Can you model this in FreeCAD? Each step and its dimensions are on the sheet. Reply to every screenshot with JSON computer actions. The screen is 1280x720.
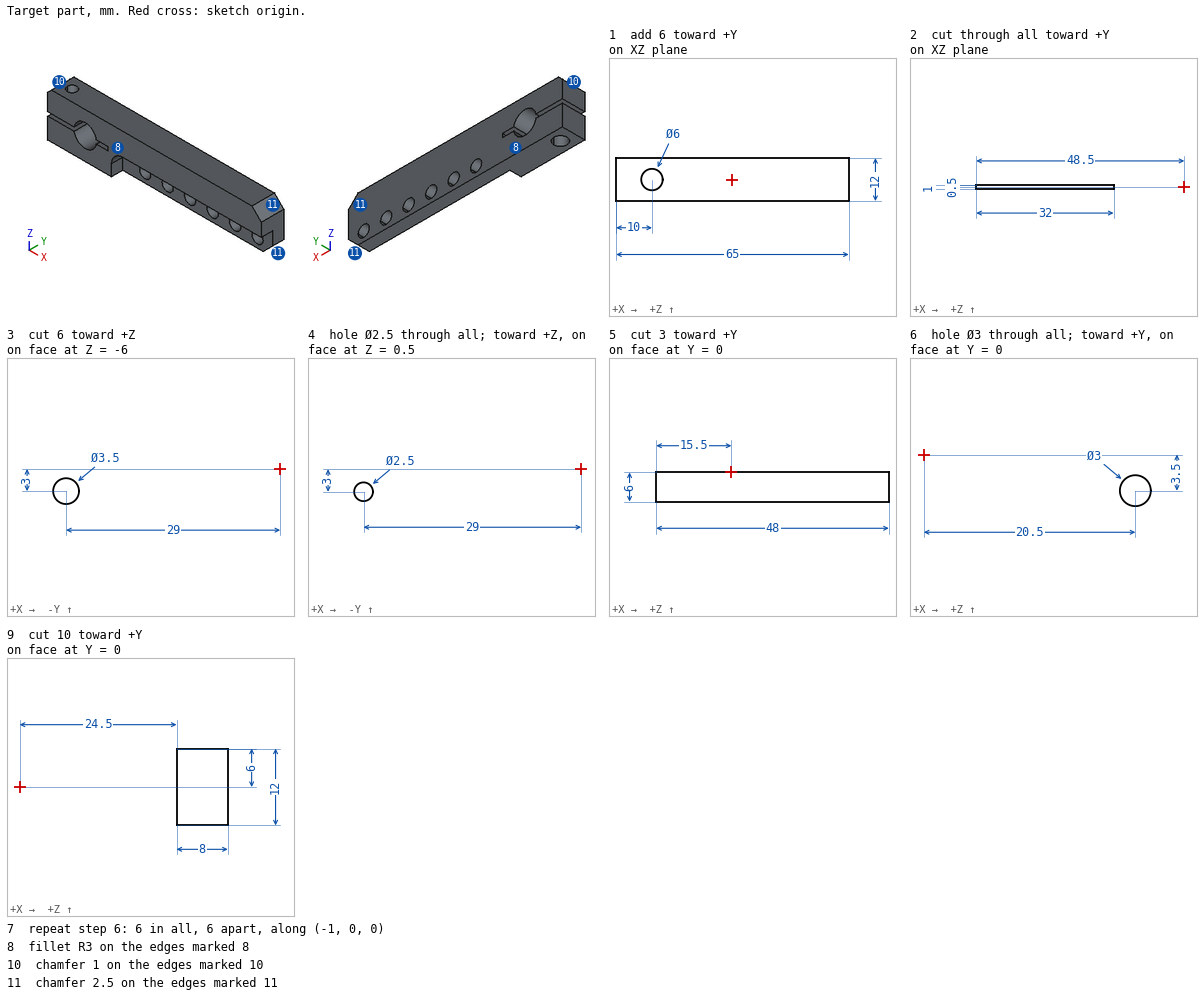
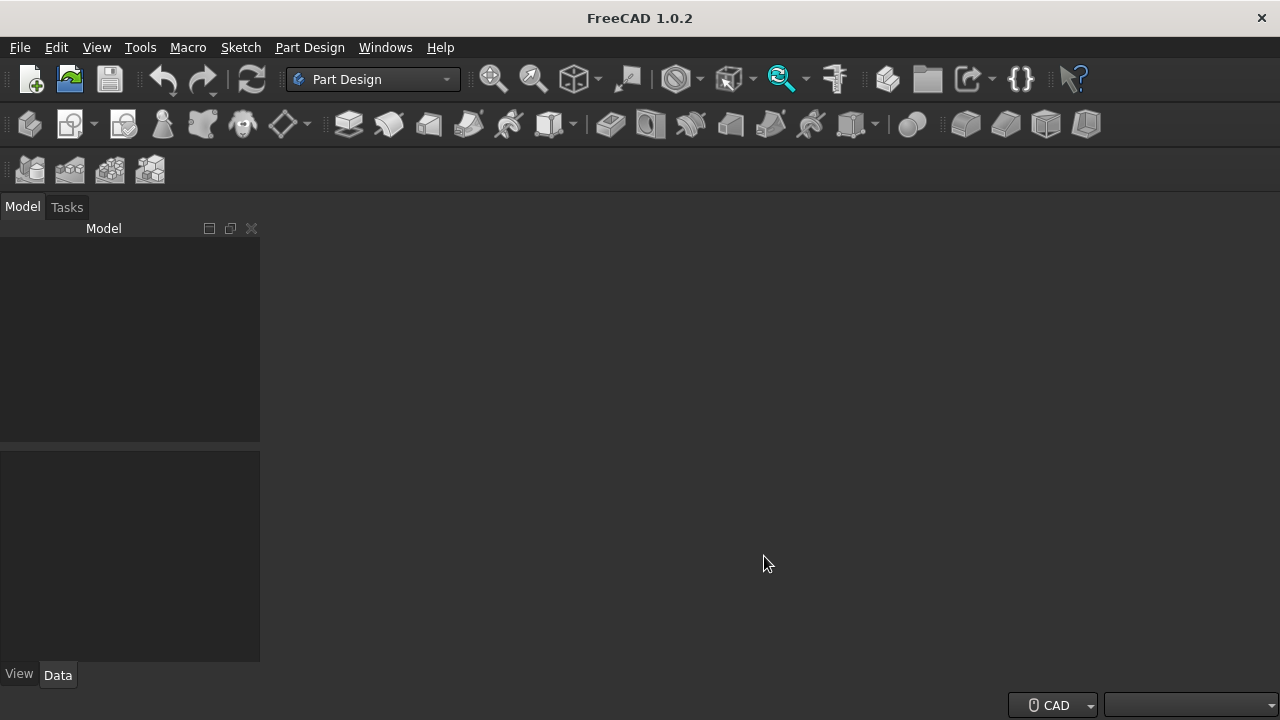
{"action": "left_click", "coordinate": [30, 80]}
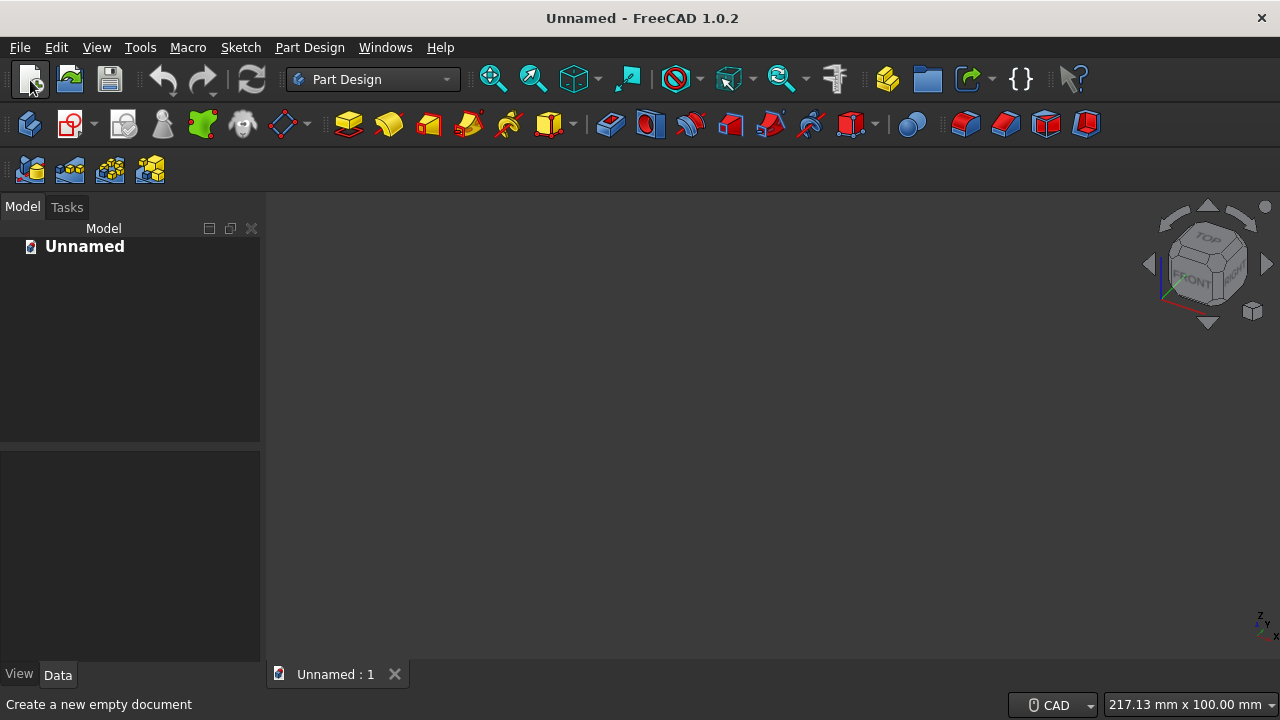
{"action": "left_click", "coordinate": [70, 124]}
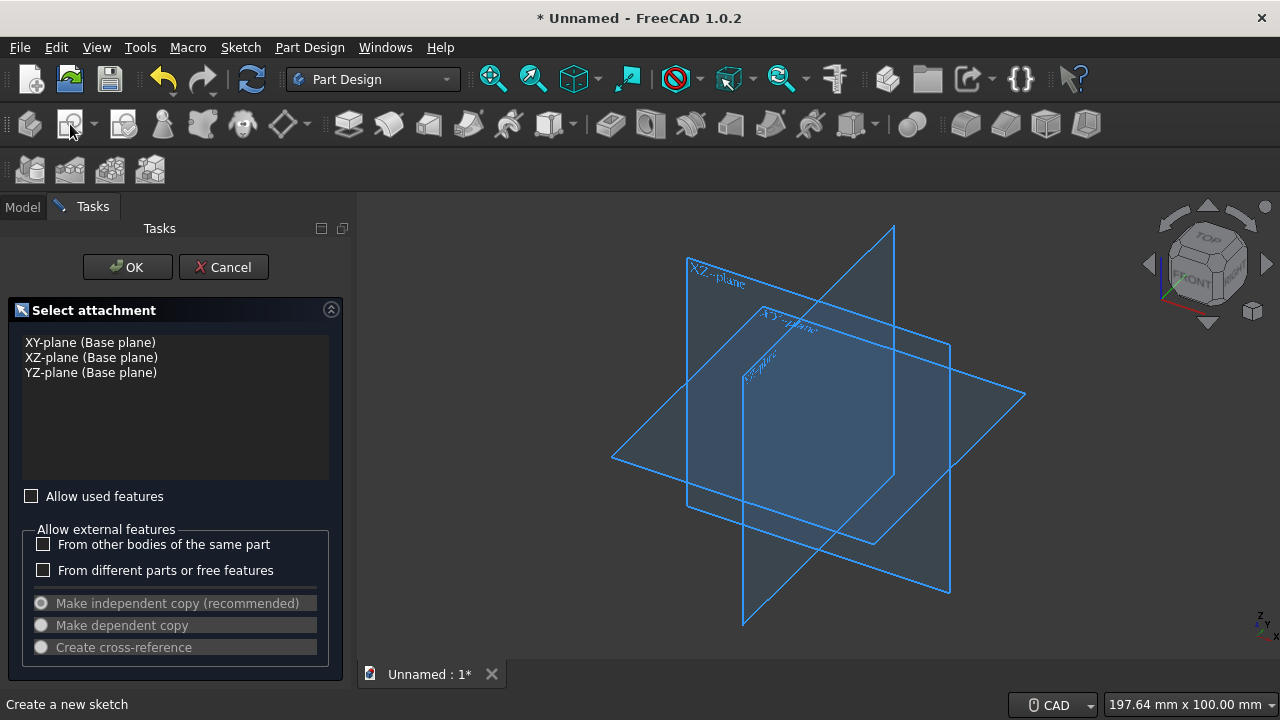
{"action": "left_click", "coordinate": [82, 358]}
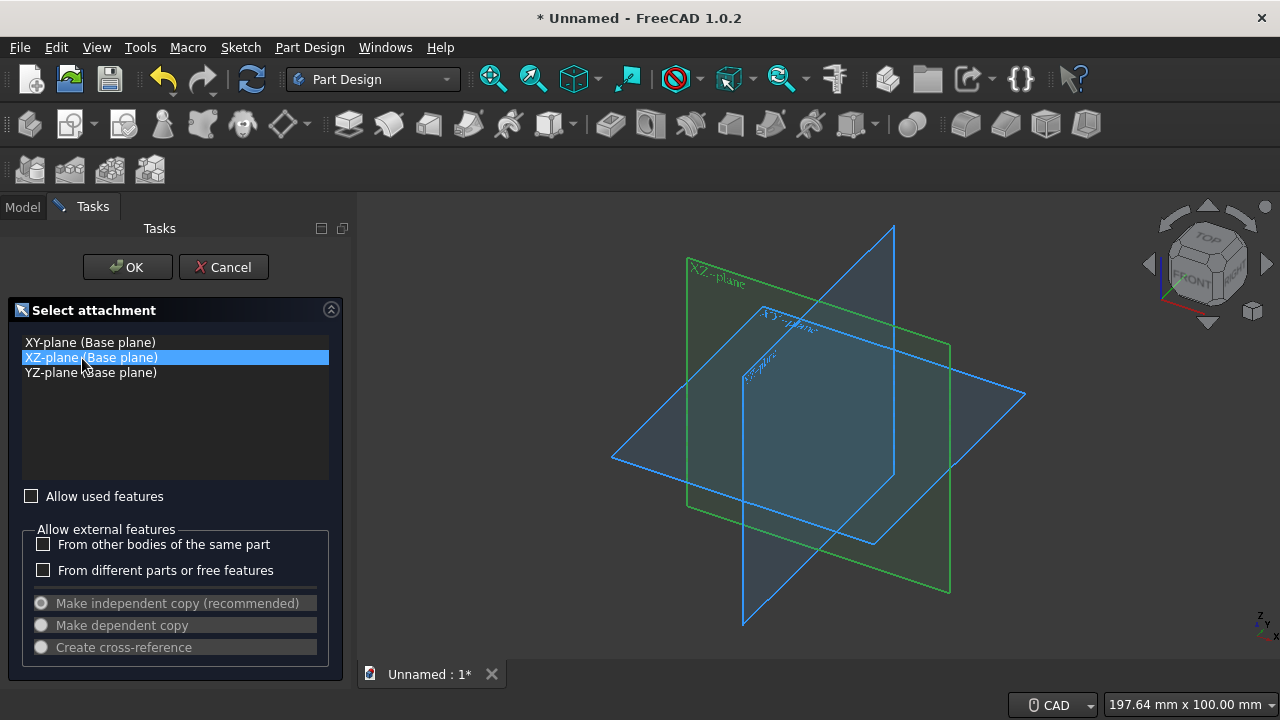
{"action": "left_click", "coordinate": [128, 267]}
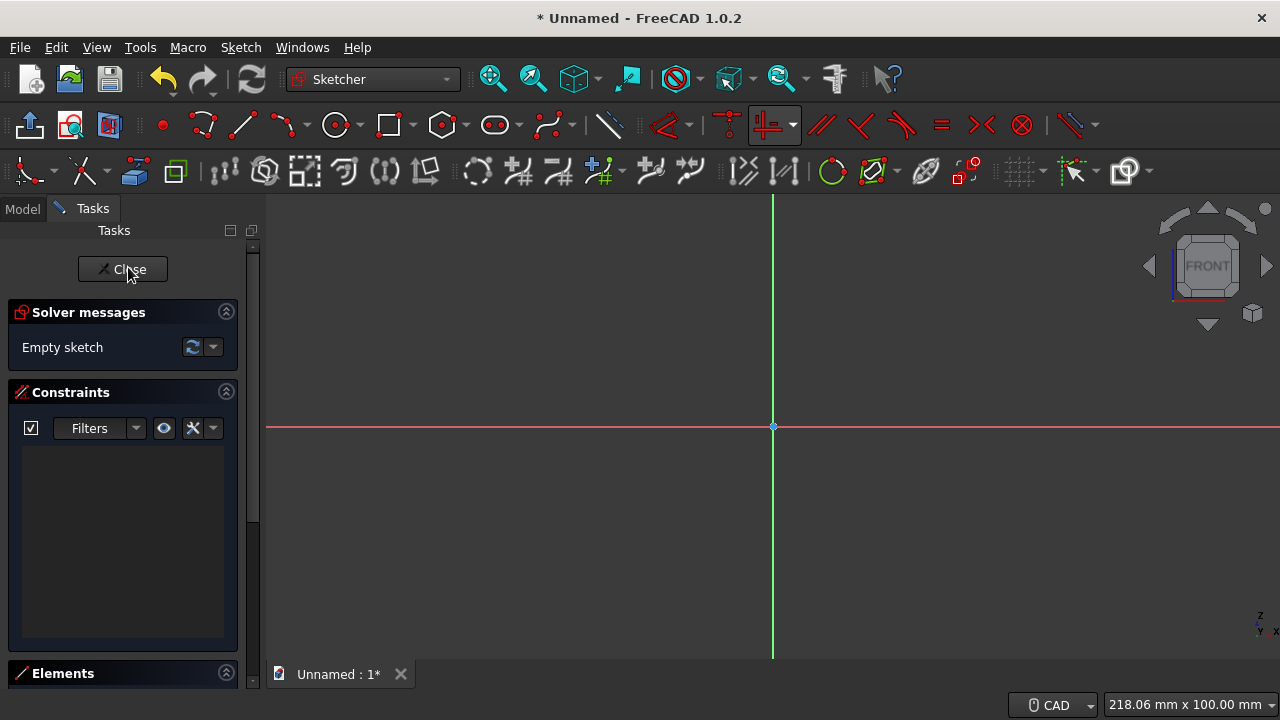
{"action": "scroll", "coordinate": [856, 426], "scroll_direction": "up", "scroll_amount": 3}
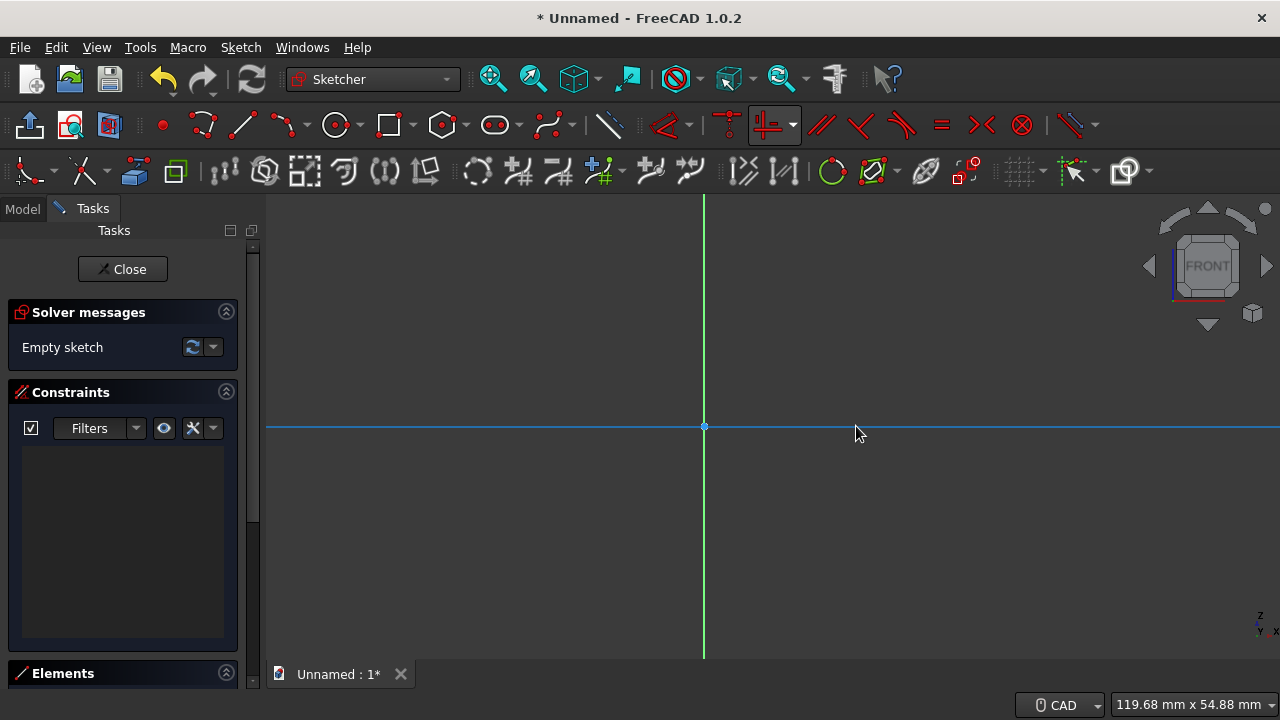
{"action": "key", "text": "g v"}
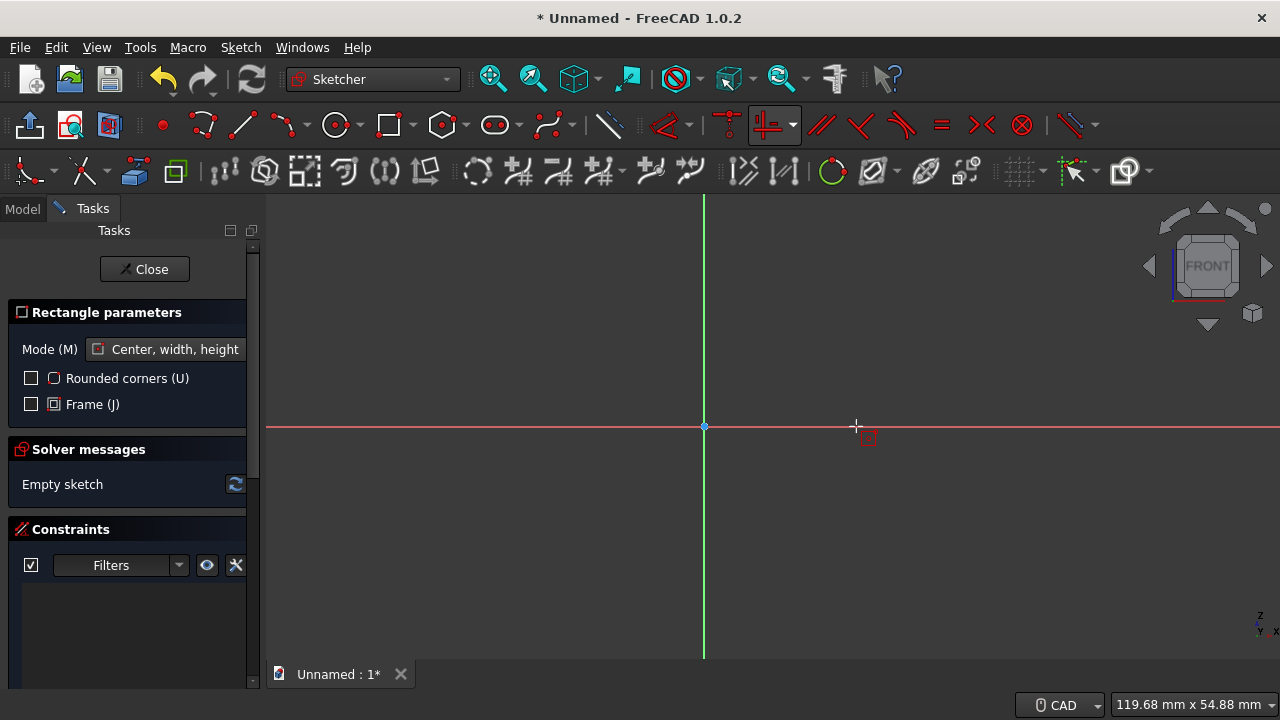
{"action": "left_click", "coordinate": [704, 426]}
{"action": "left_click", "coordinate": [980, 376]}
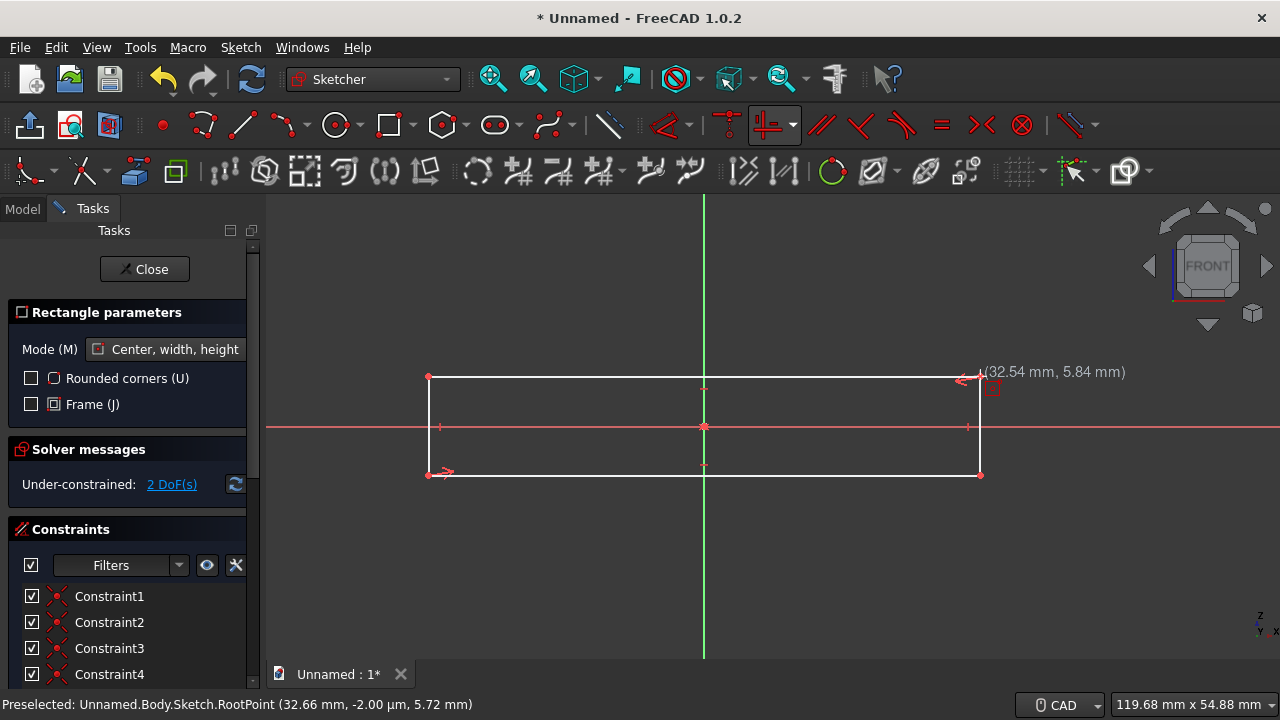
{"action": "left_click", "coordinate": [336, 126]}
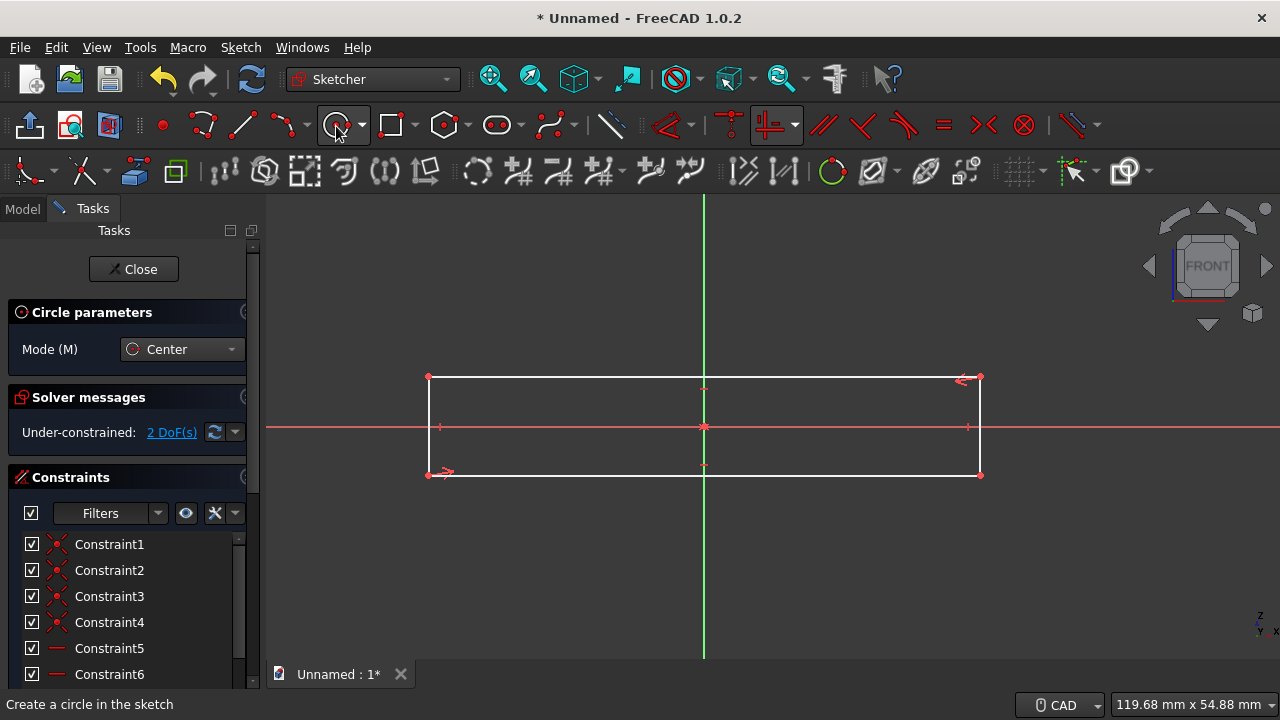
{"action": "left_click", "coordinate": [514, 426]}
{"action": "left_click", "coordinate": [532, 409]}
{"action": "key", "text": "Escape"}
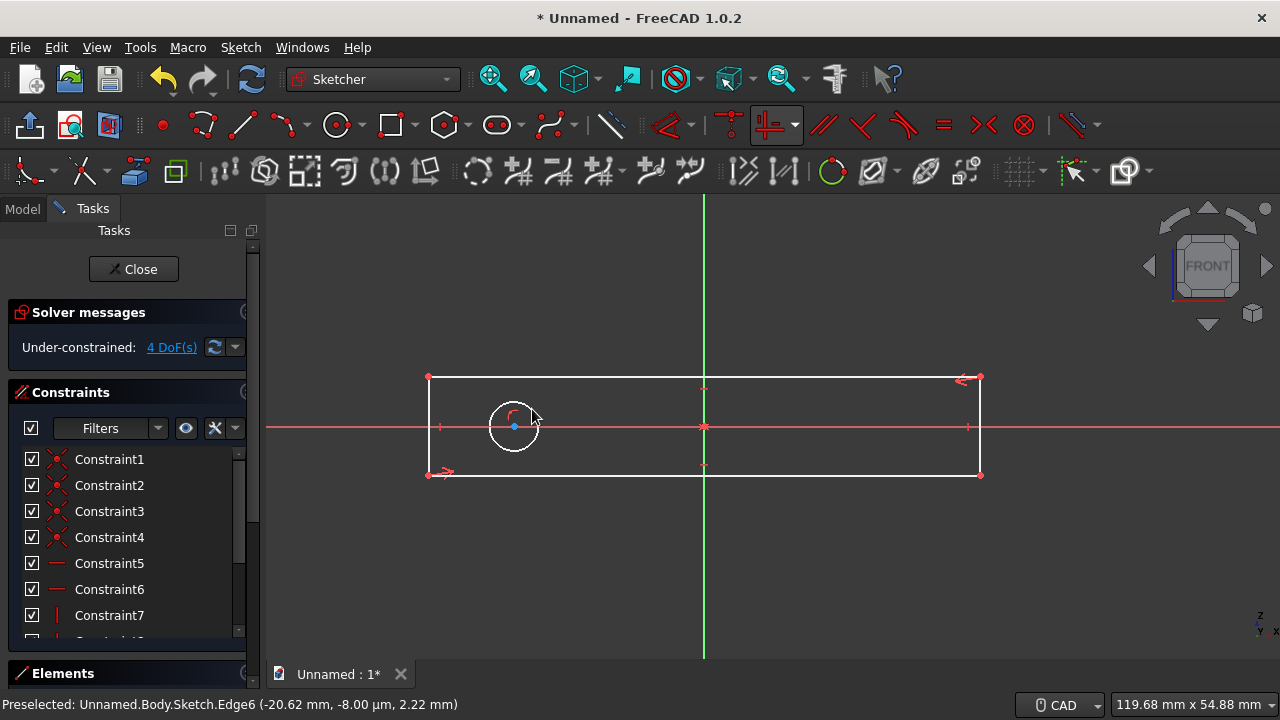
{"action": "left_click", "coordinate": [666, 126]}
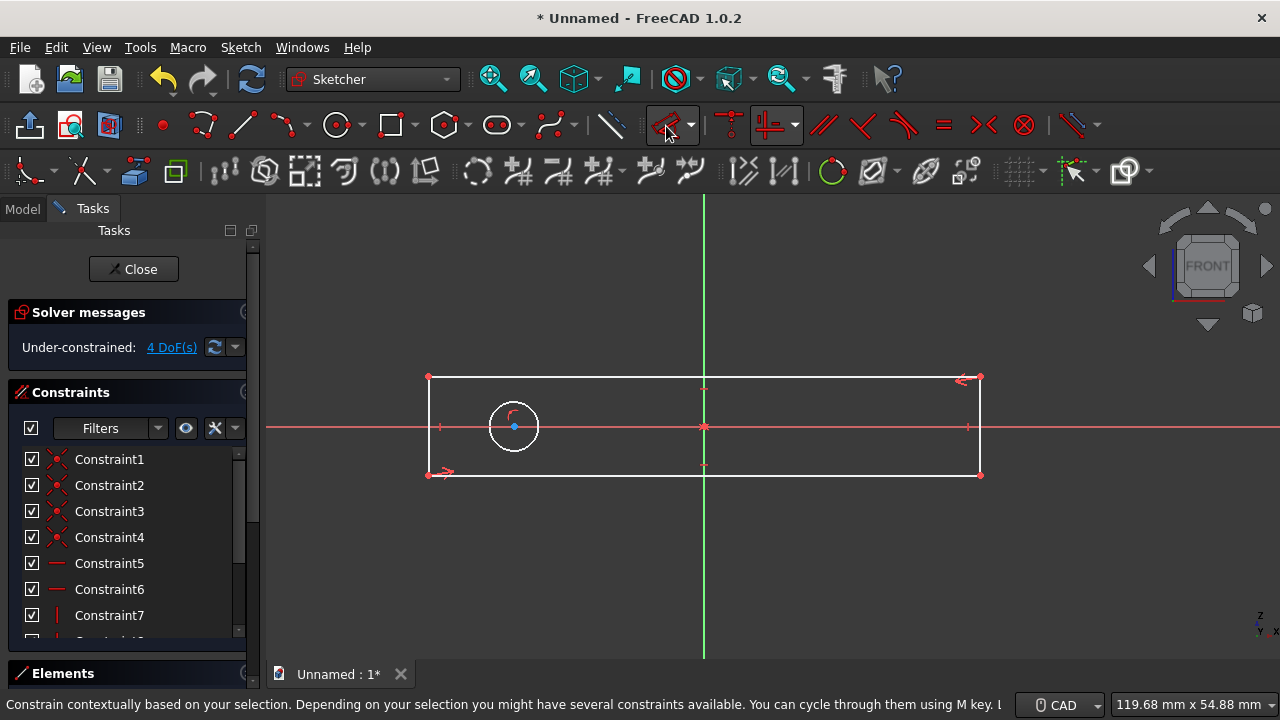
{"action": "left_click", "coordinate": [531, 409]}
{"action": "left_click", "coordinate": [568, 410]}